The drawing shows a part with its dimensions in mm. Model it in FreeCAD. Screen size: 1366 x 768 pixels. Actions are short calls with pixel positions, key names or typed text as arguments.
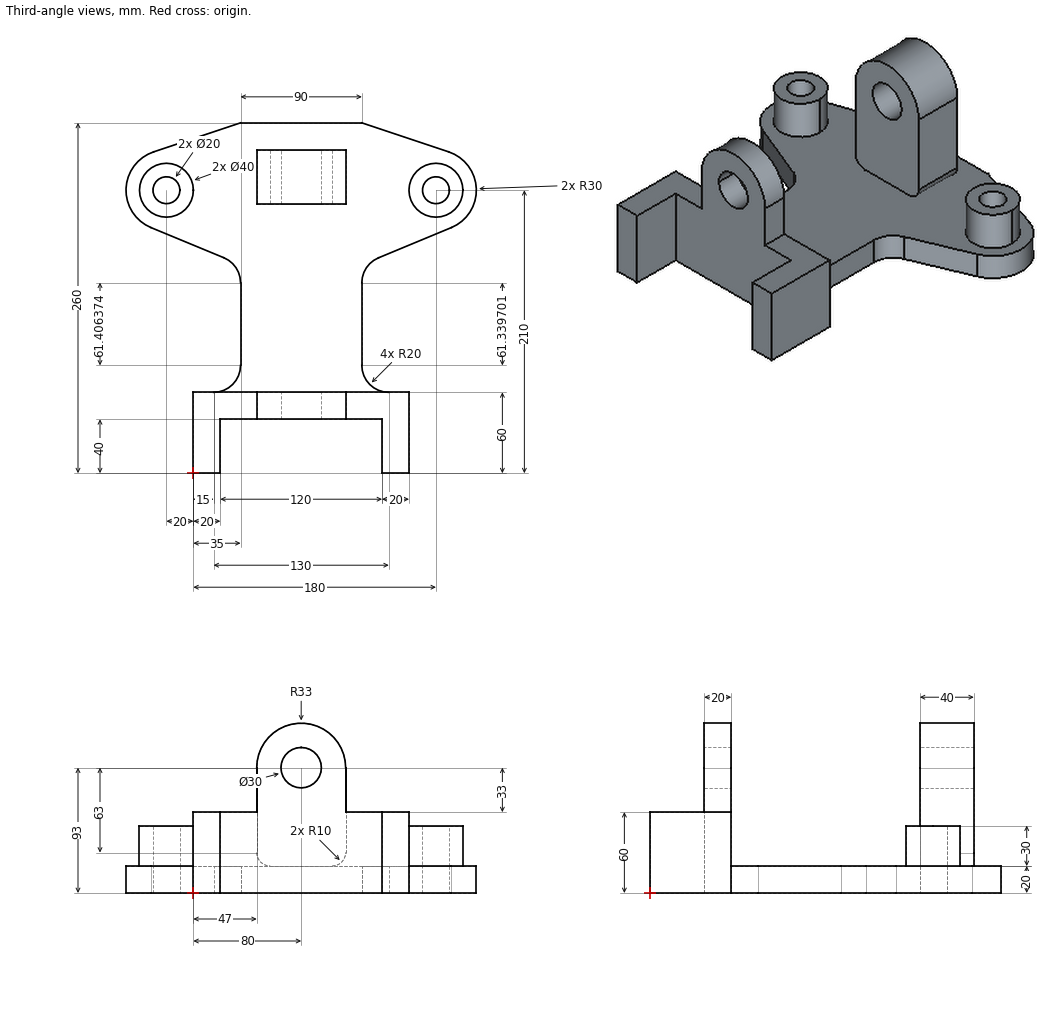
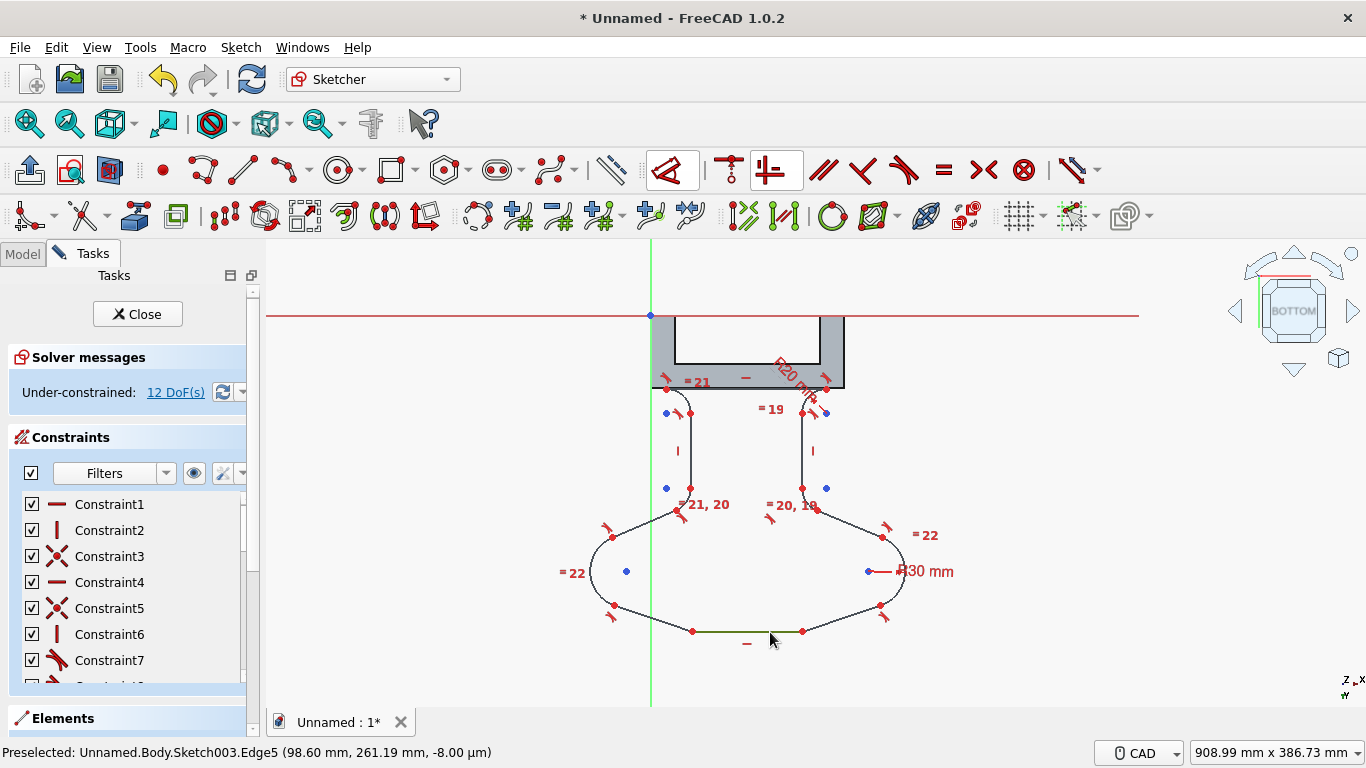
key(l)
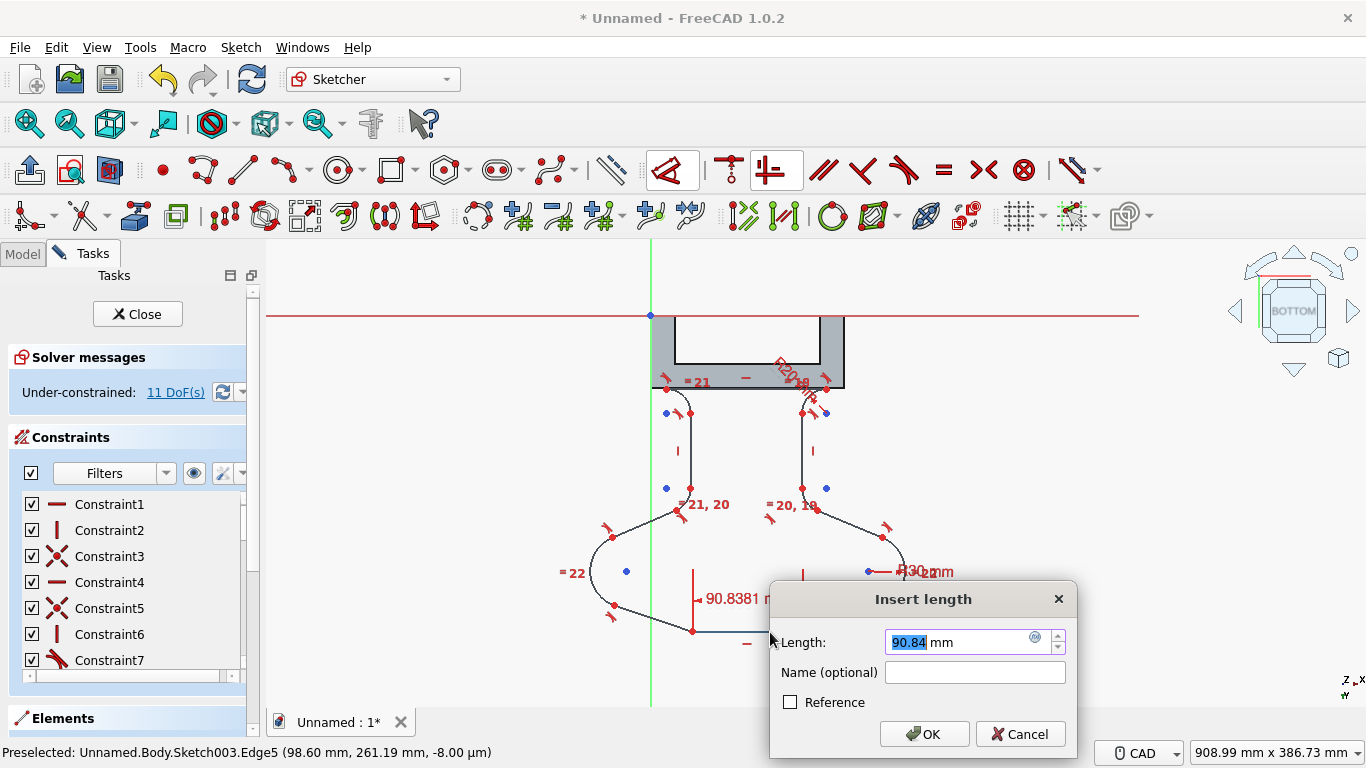
text(90)
key(Return)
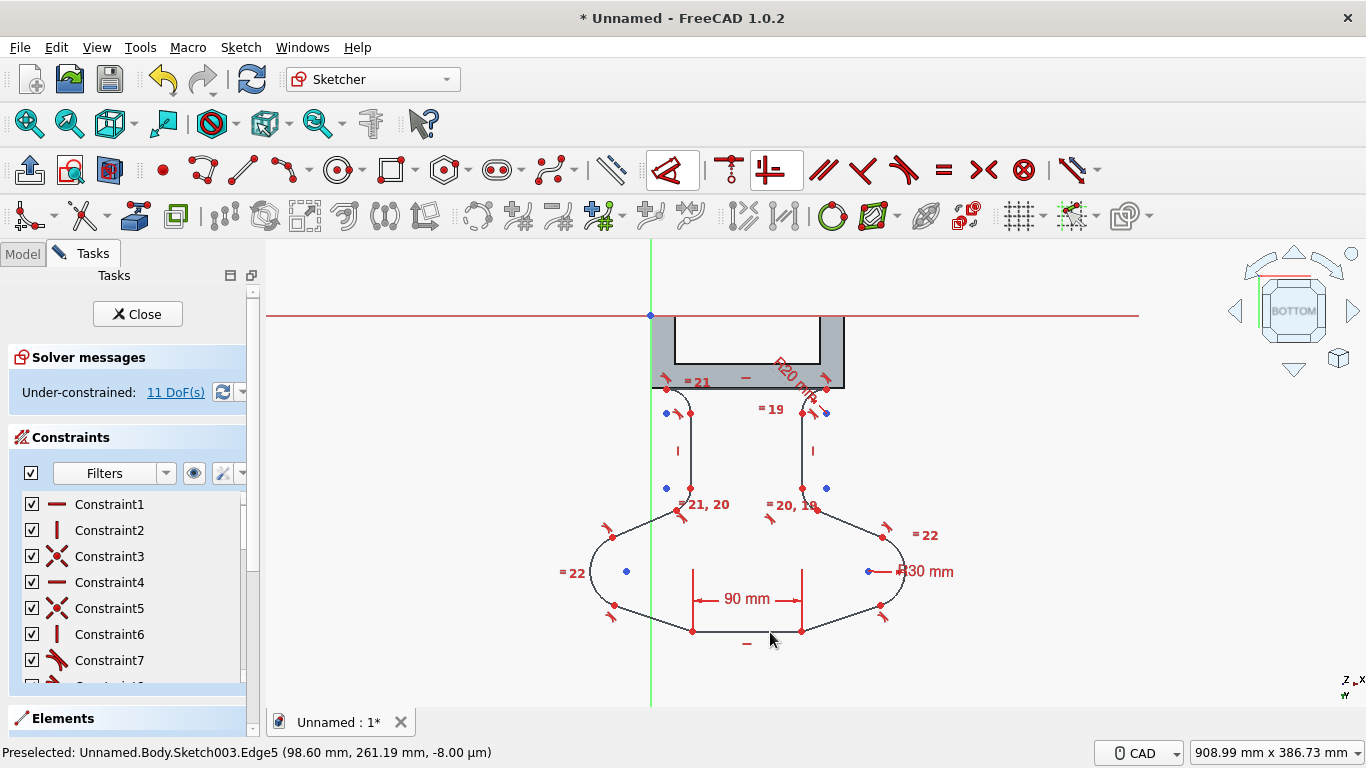
click(714, 389)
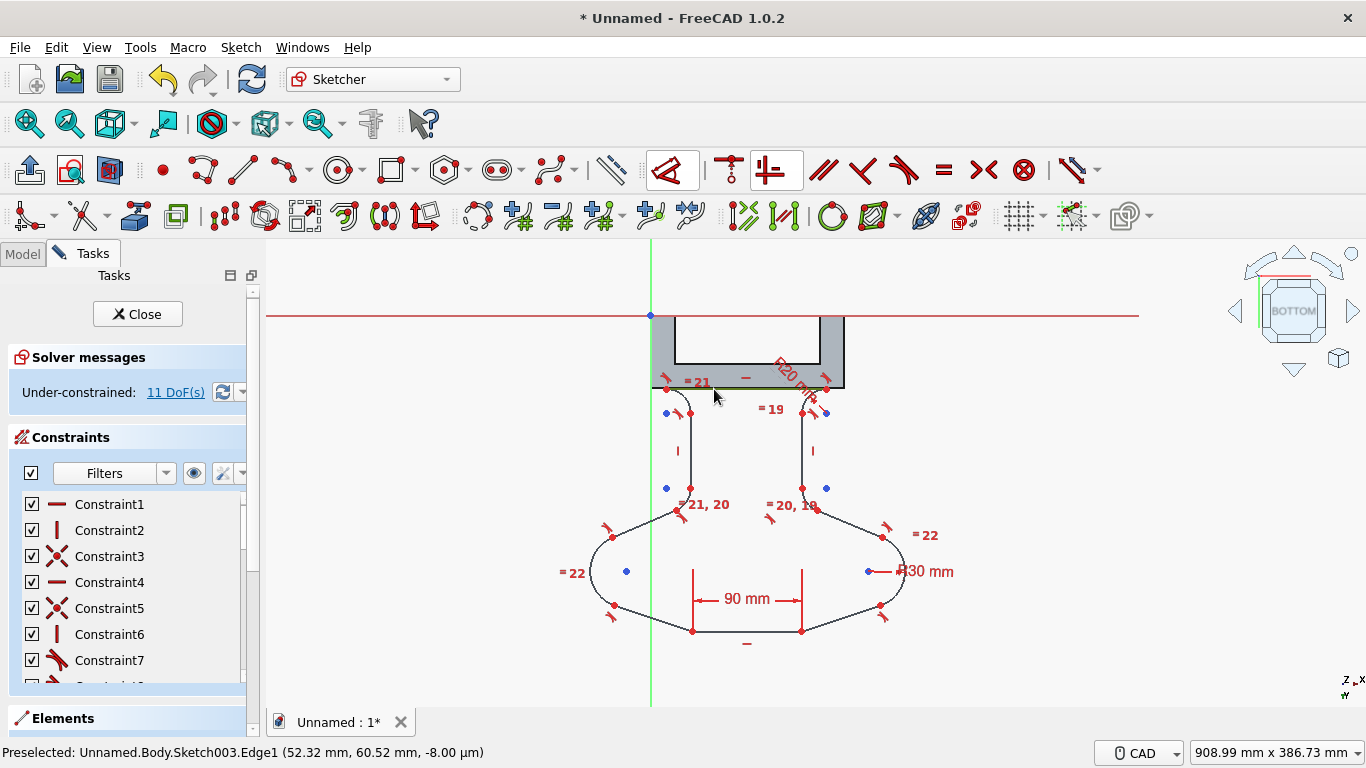
key(l)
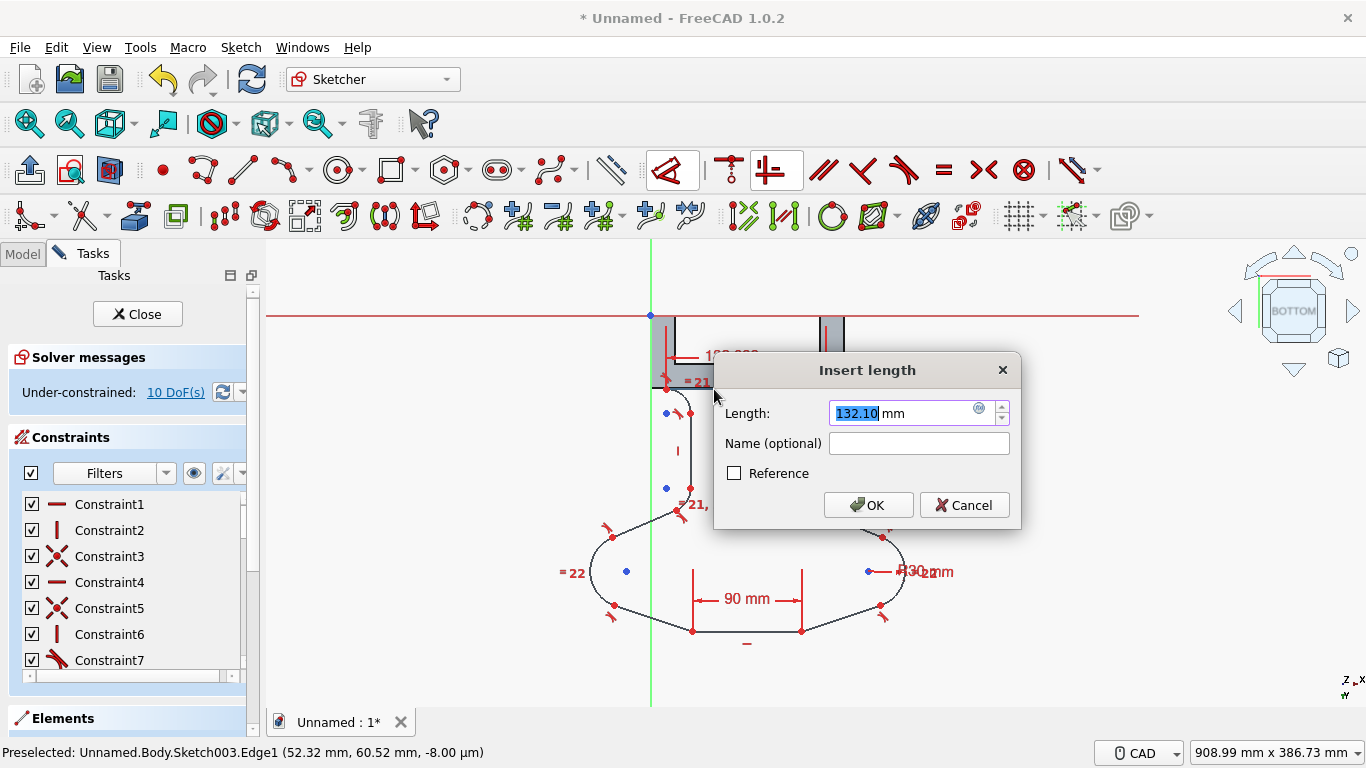
text(130)
key(Return)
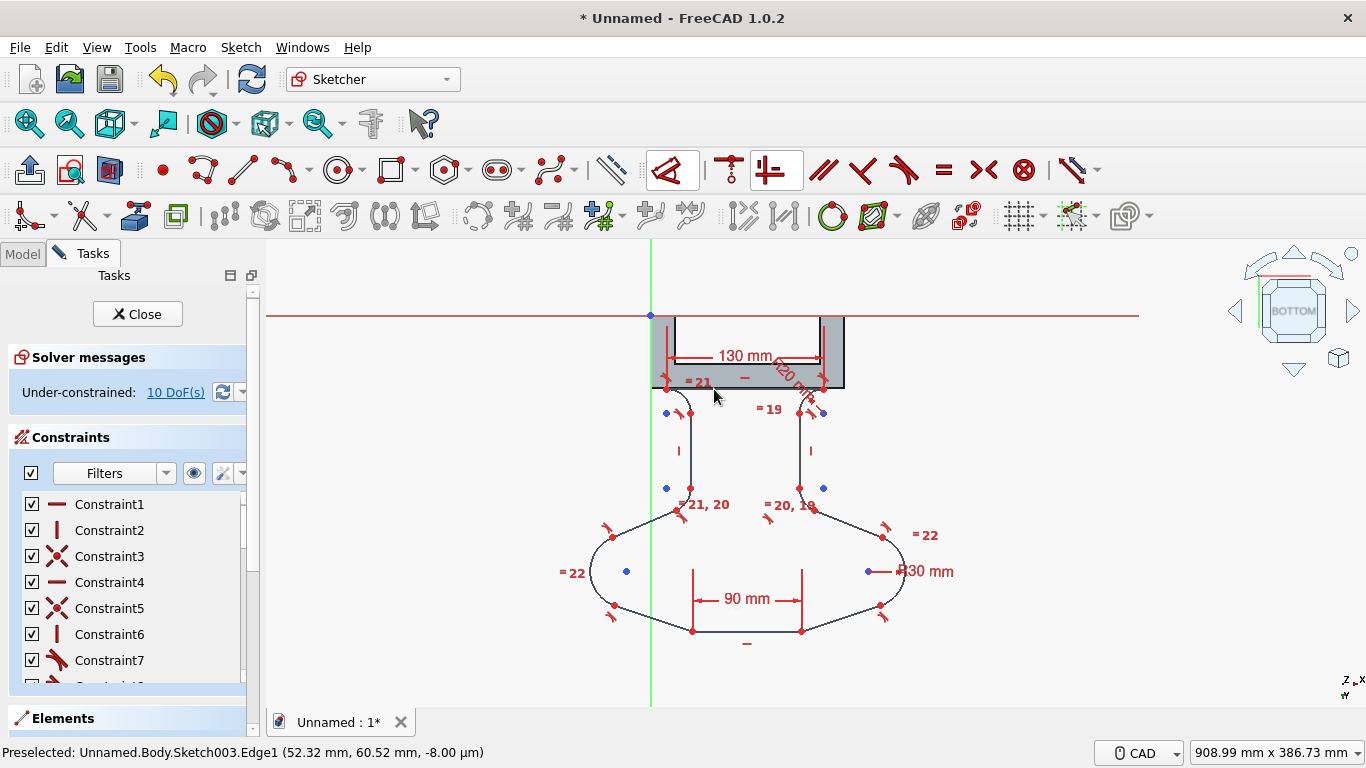
scroll(667, 389, up, 4)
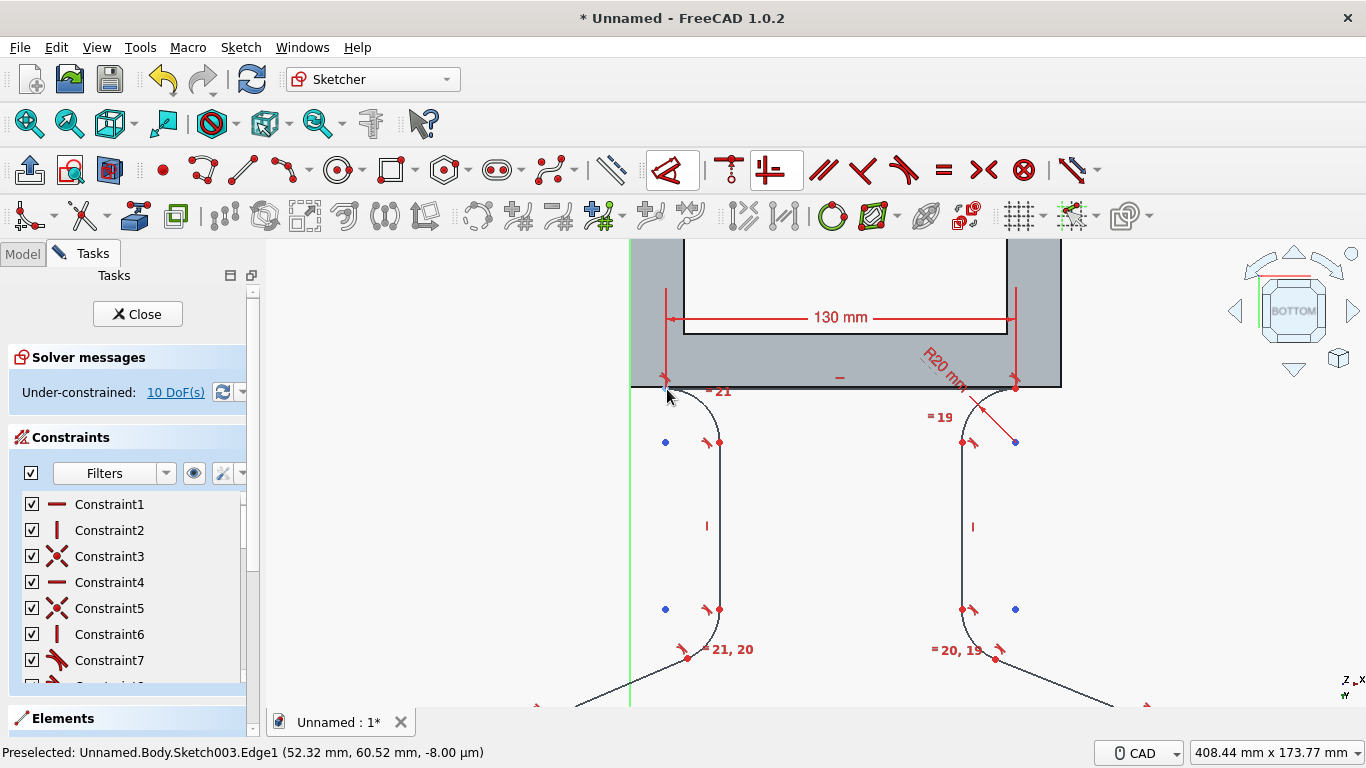
click(666, 389)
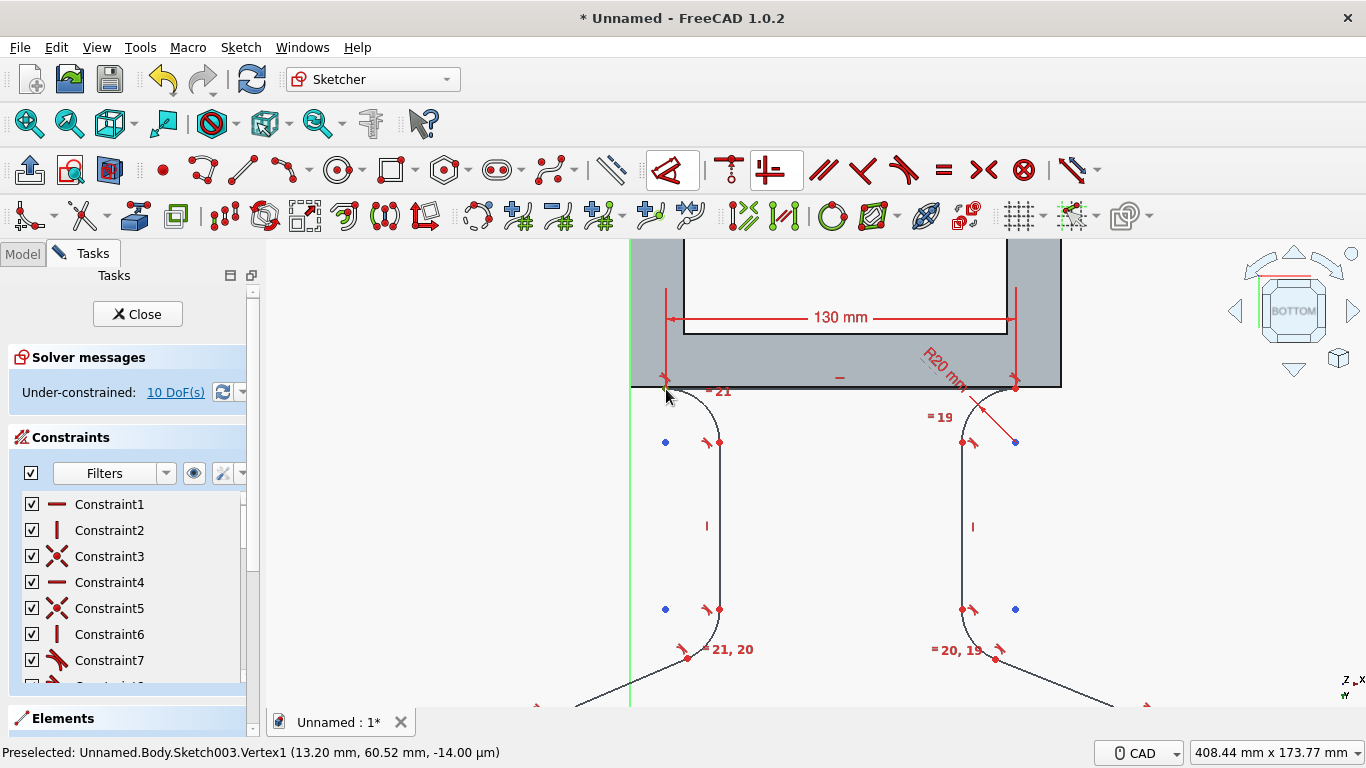
key(l)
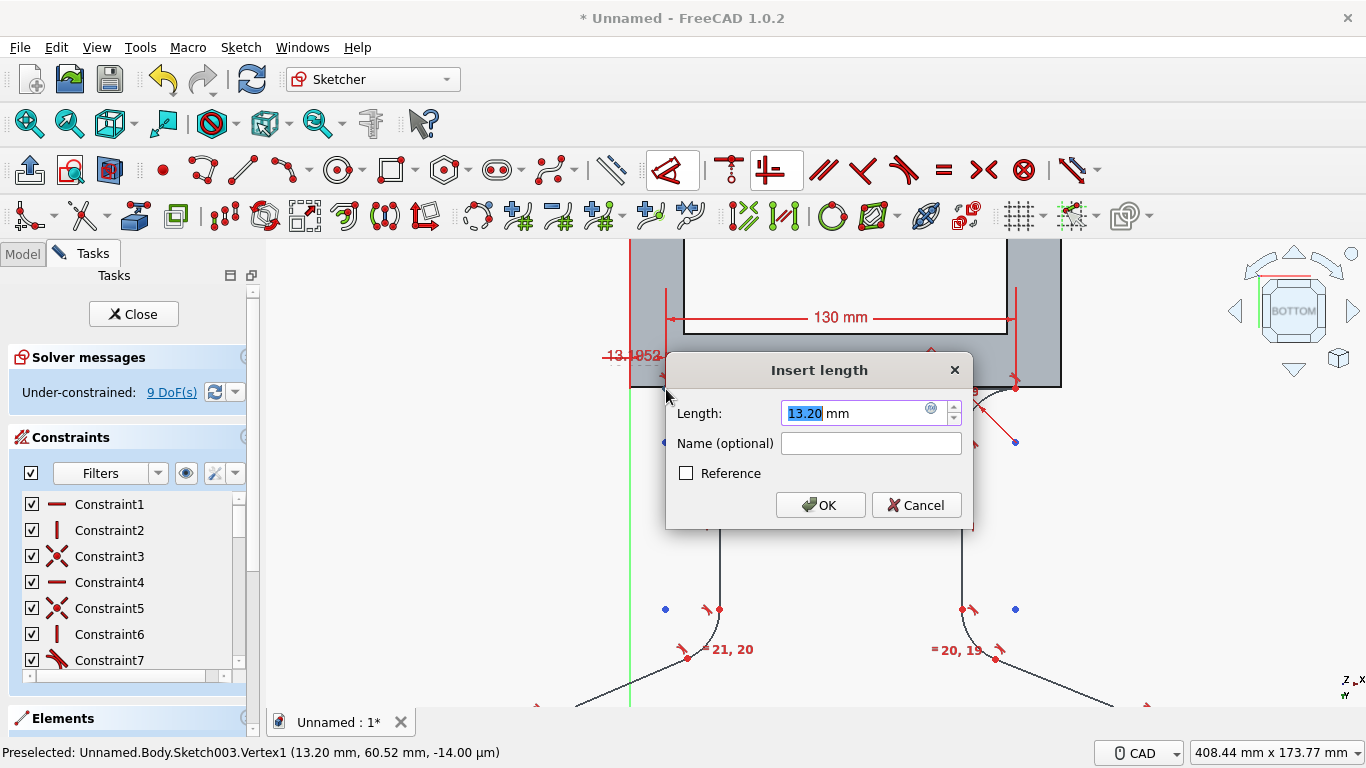
text(15)
key(Return)